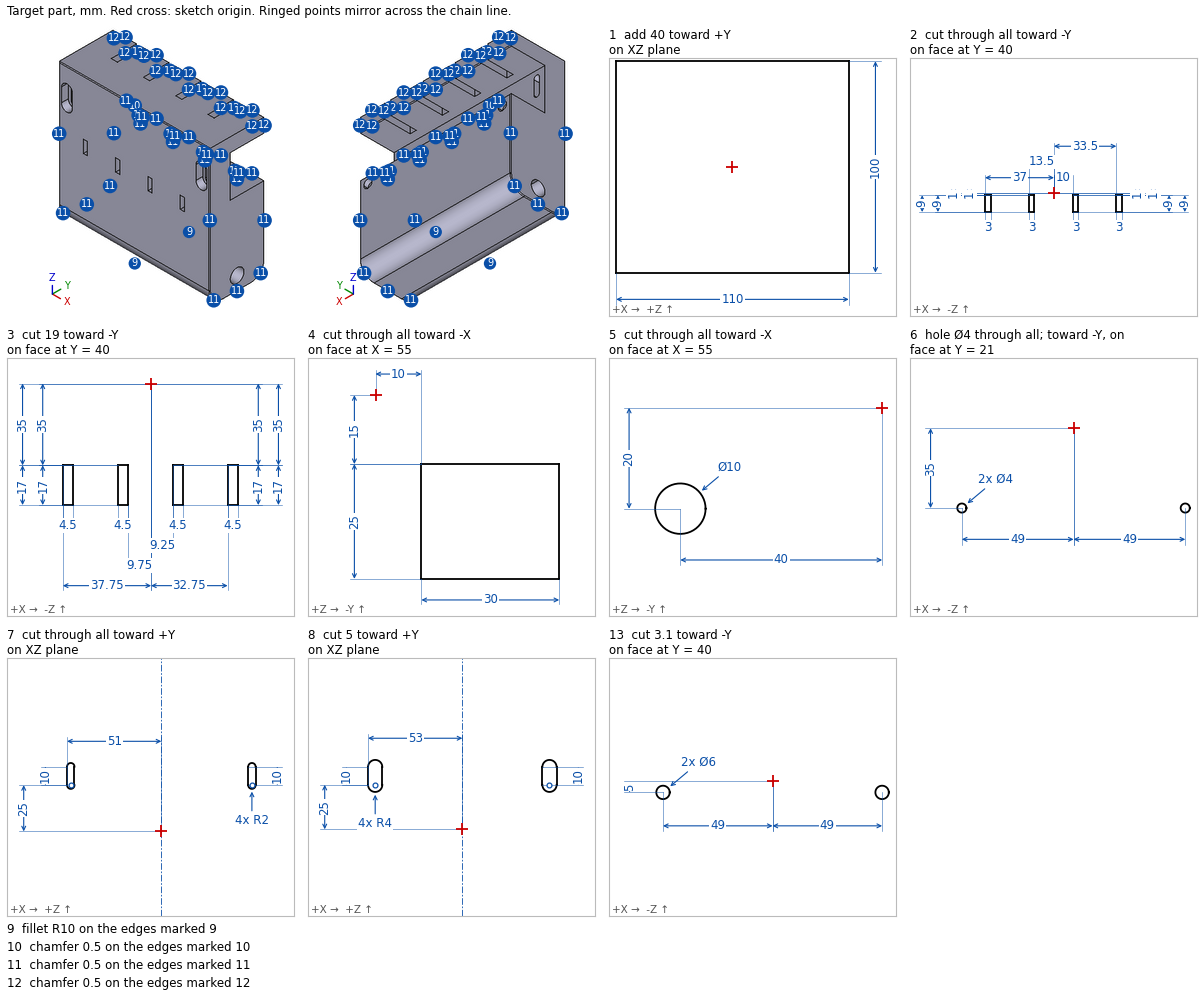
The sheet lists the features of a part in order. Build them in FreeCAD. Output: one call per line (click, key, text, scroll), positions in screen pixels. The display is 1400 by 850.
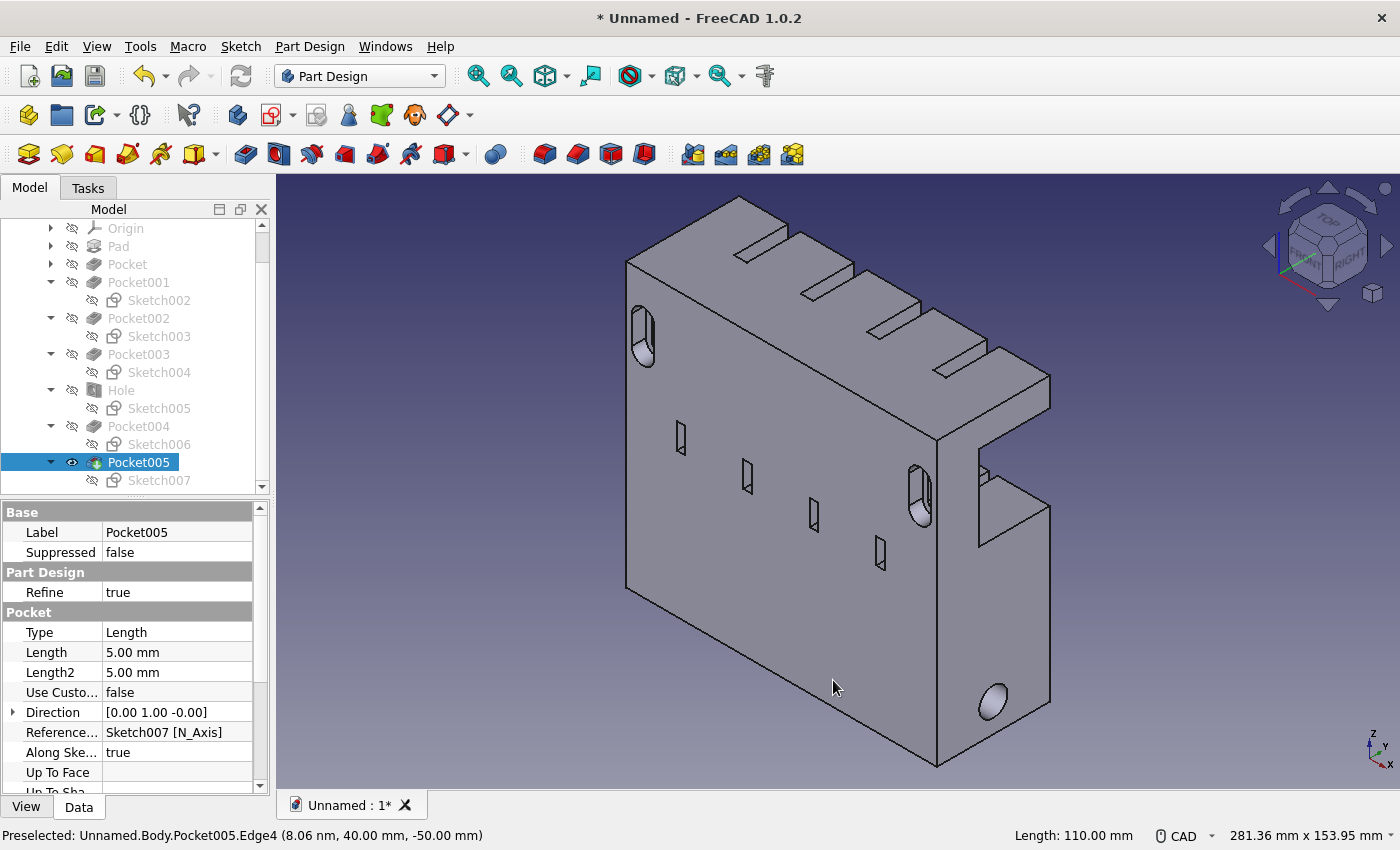
key(2)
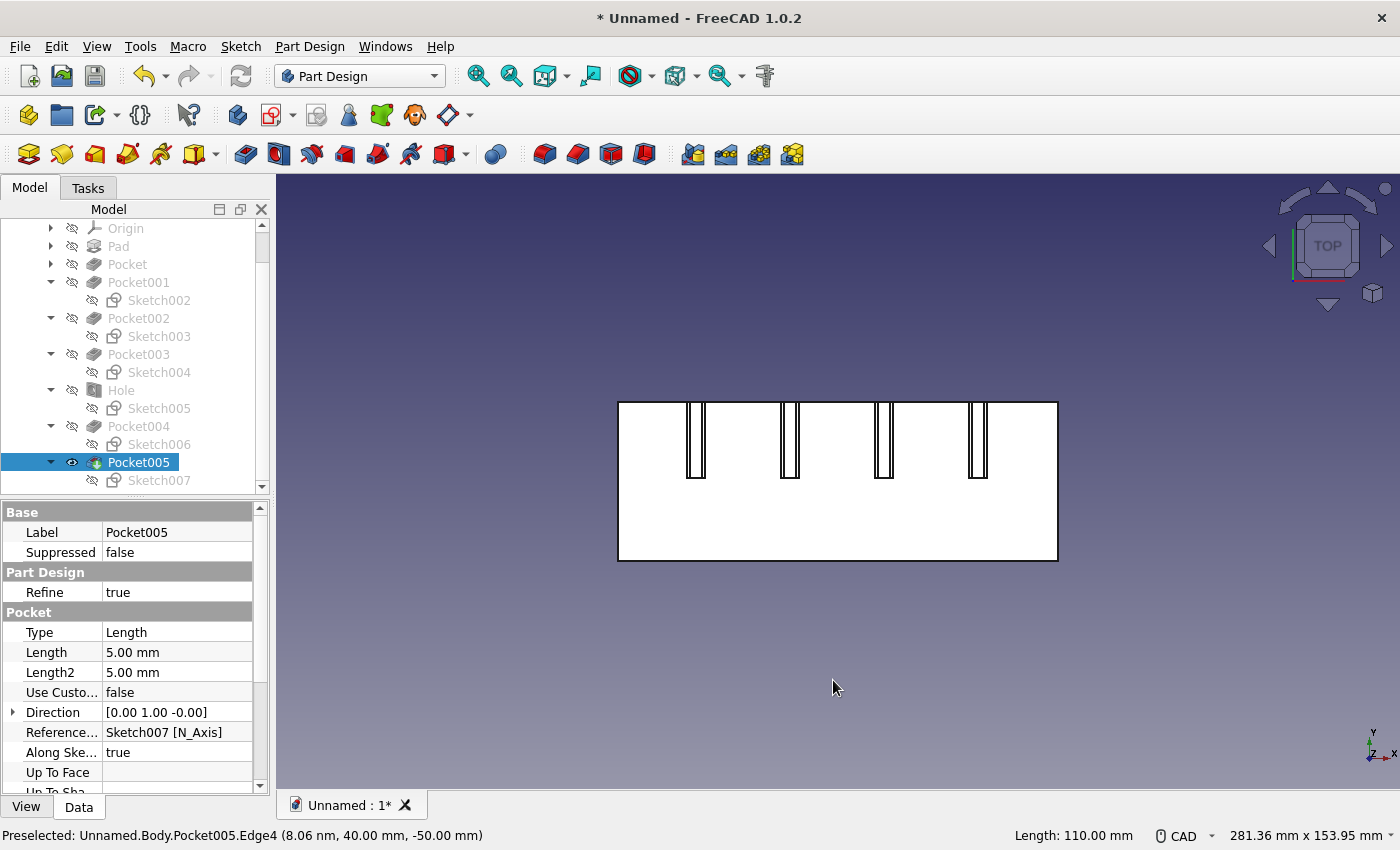
key(v)
key(f)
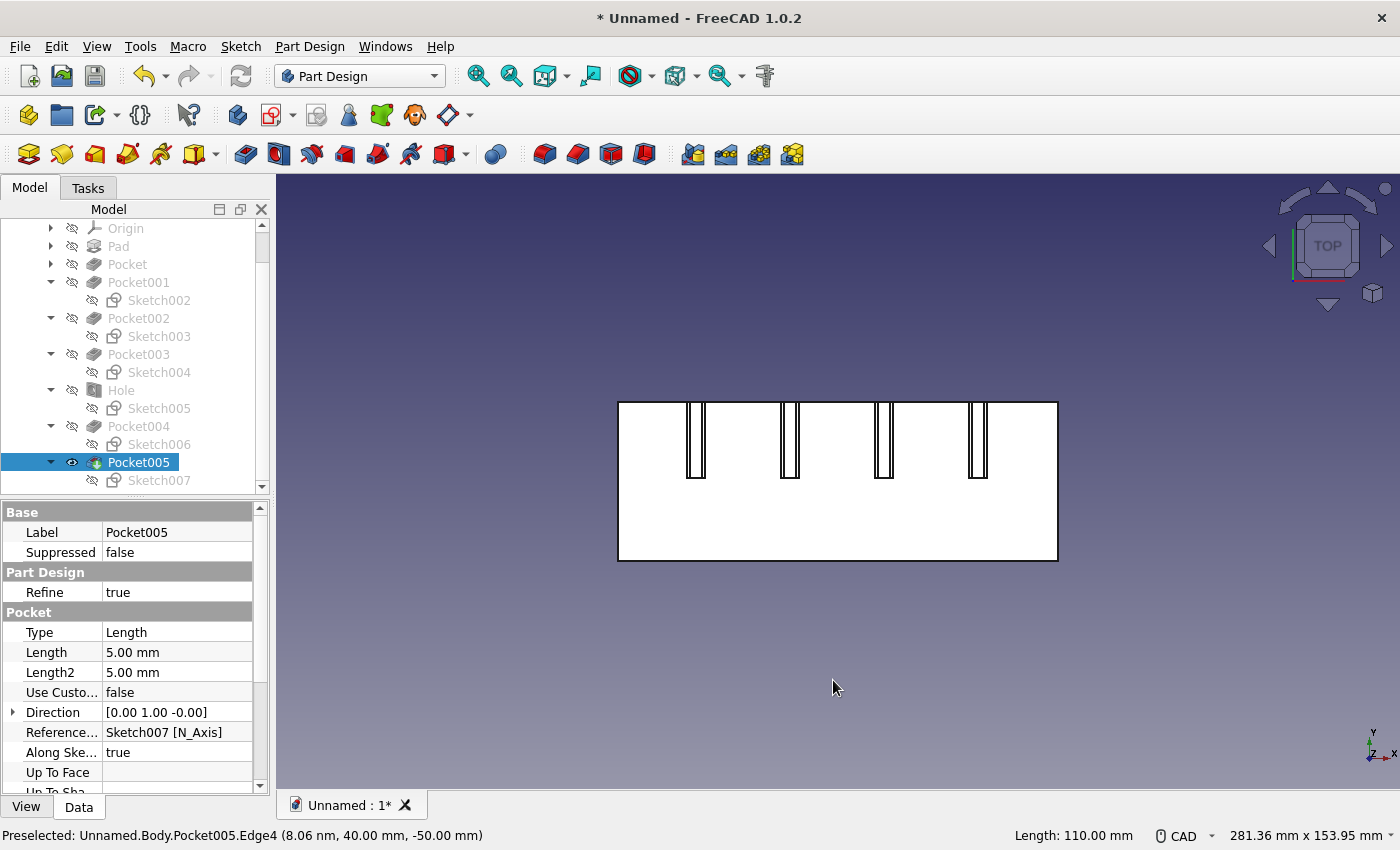
key(1)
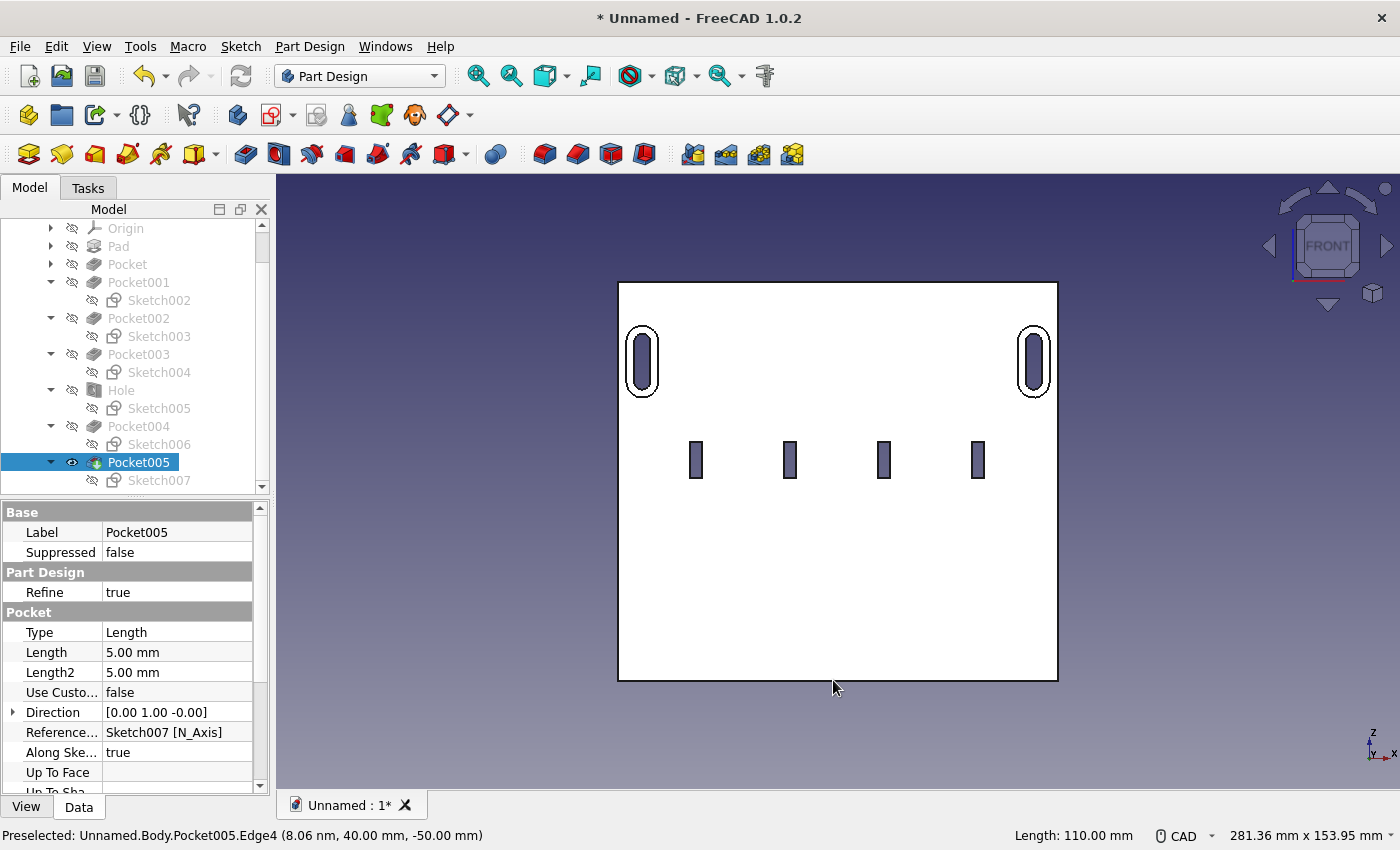
key(3)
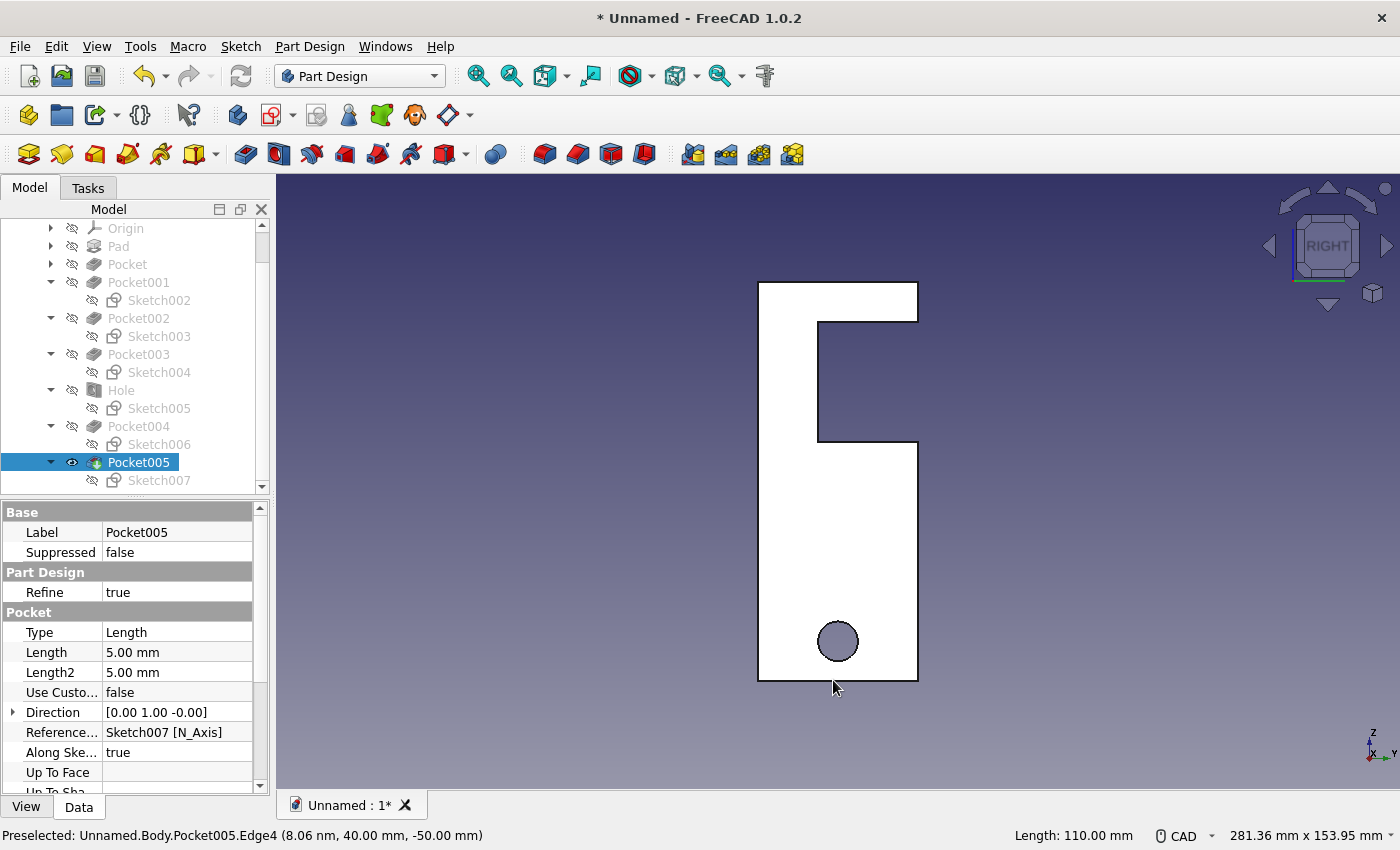
key(5)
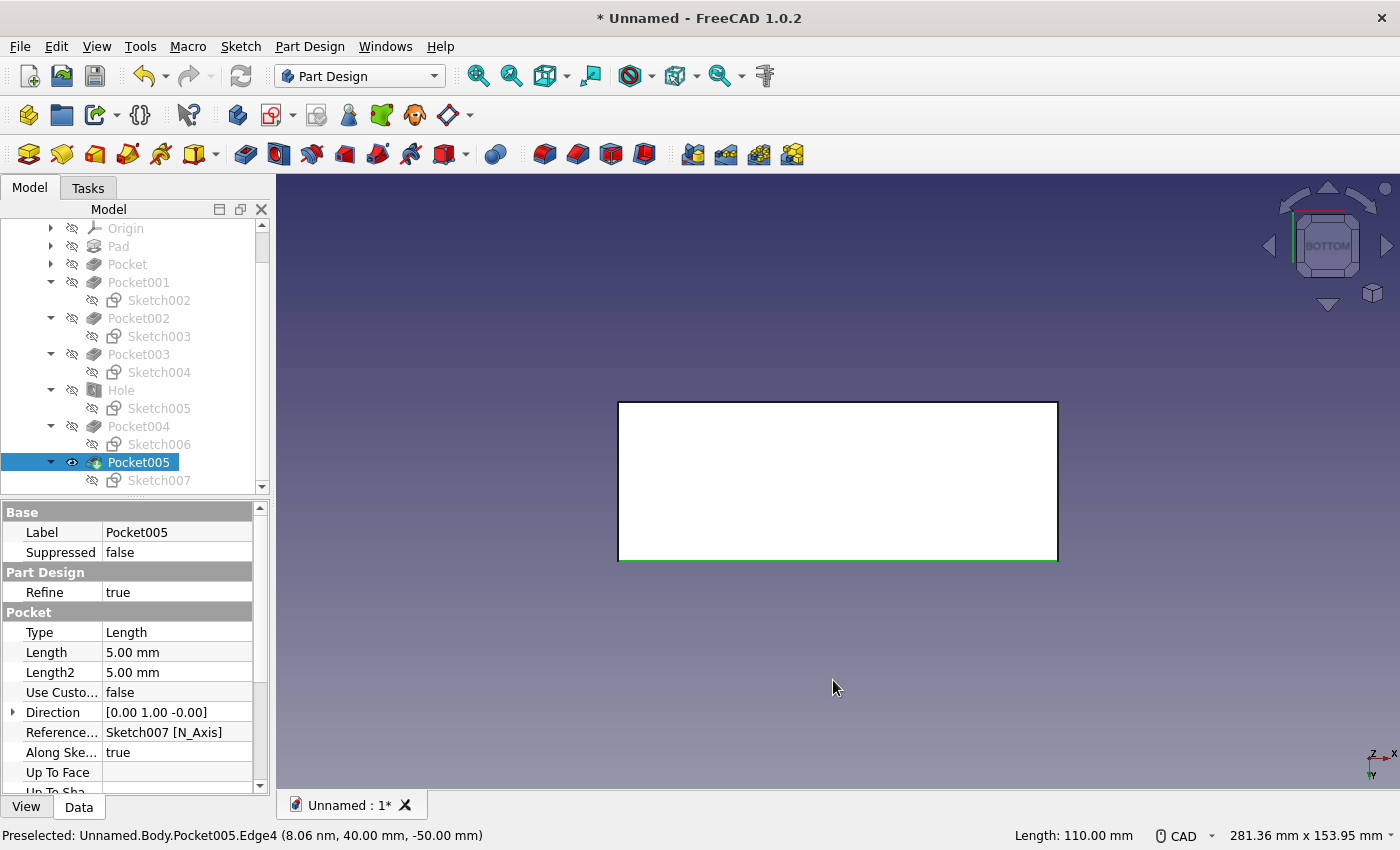
key(v)
key(f)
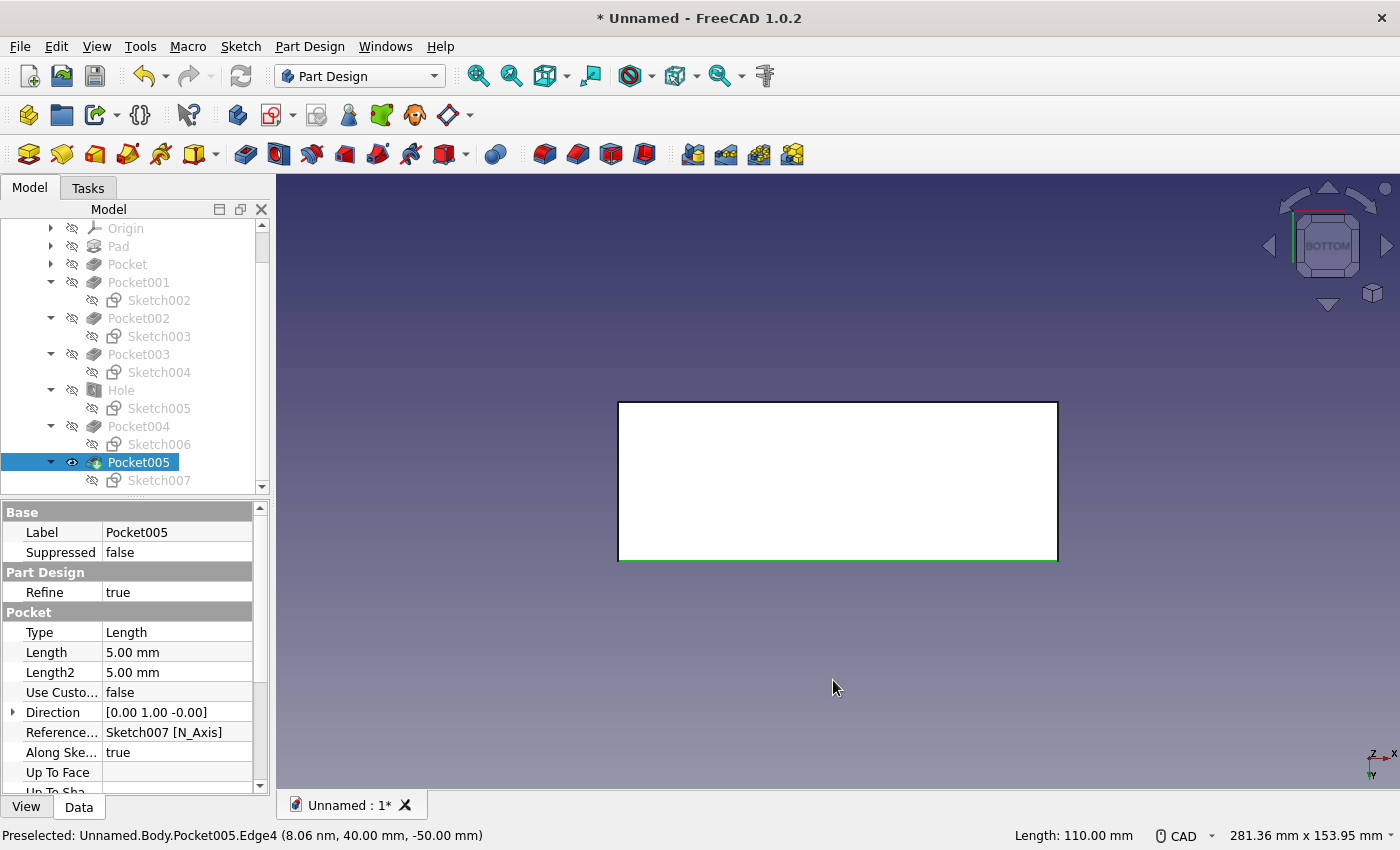
click(838, 401, ctrl)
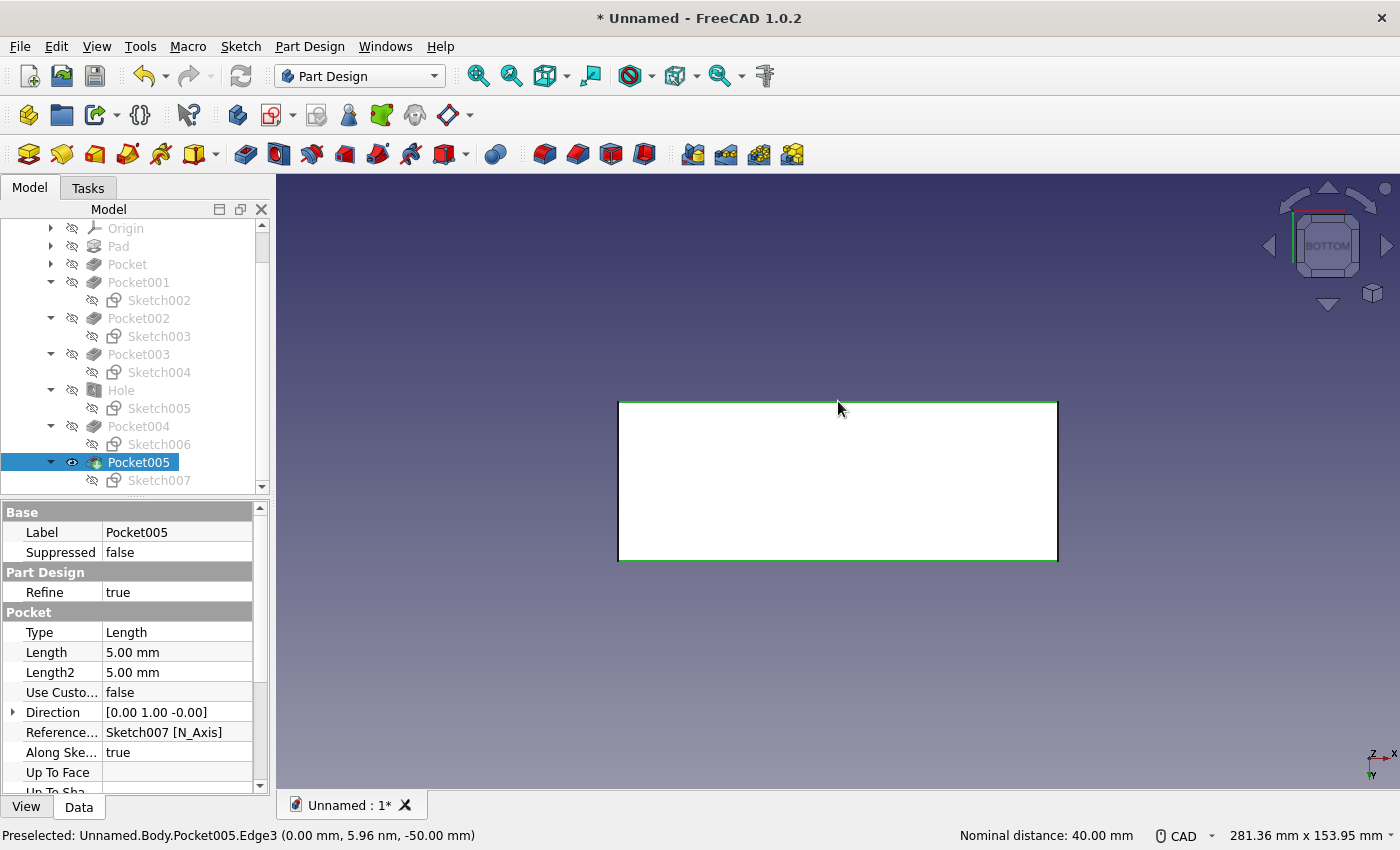
click(545, 154)